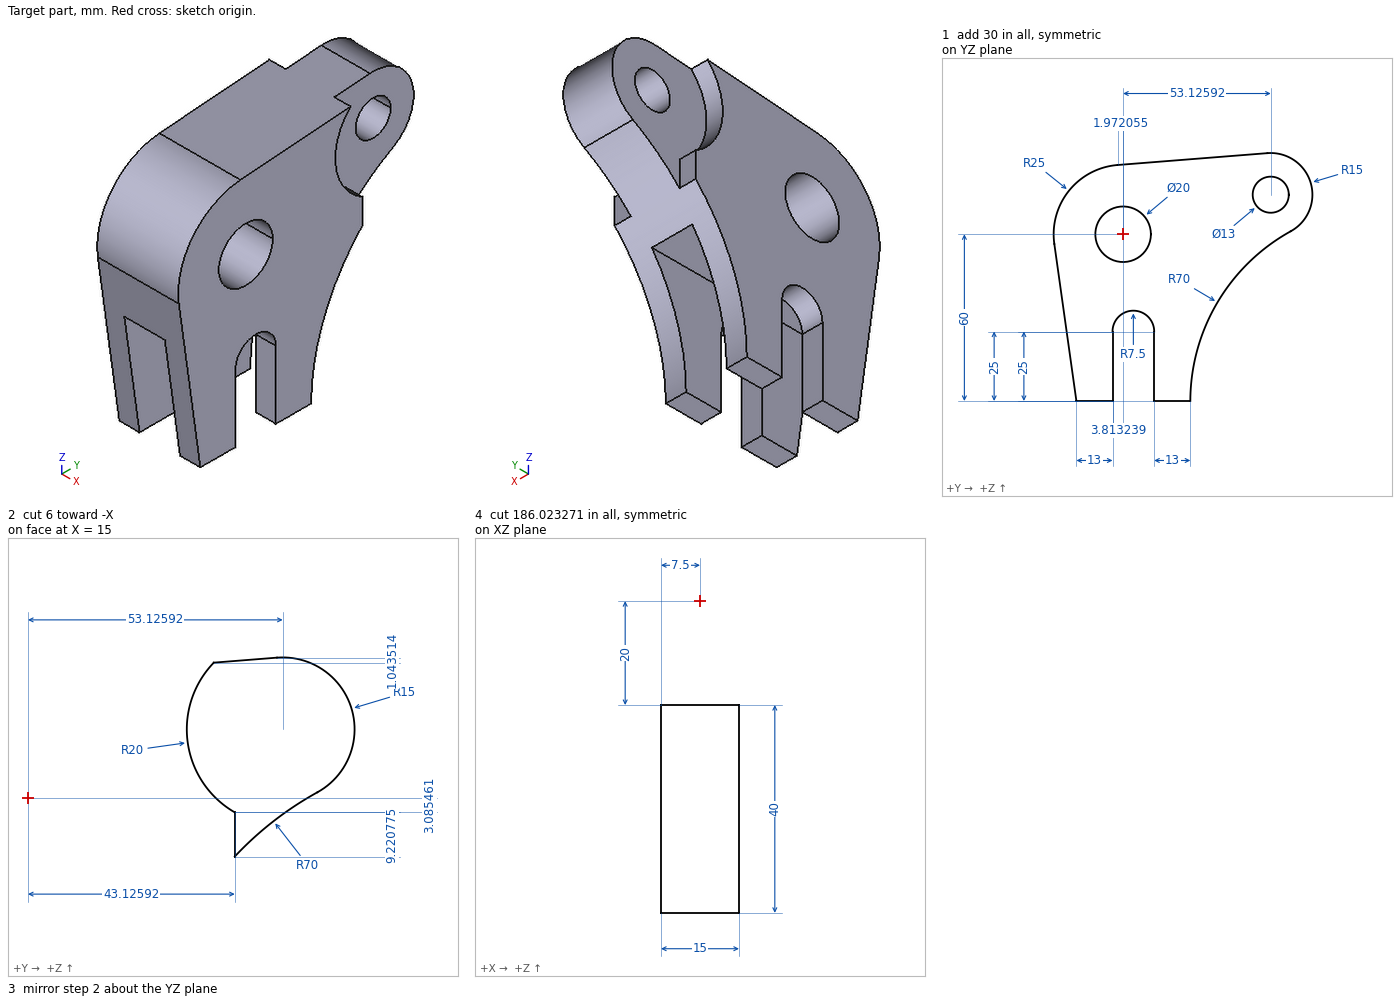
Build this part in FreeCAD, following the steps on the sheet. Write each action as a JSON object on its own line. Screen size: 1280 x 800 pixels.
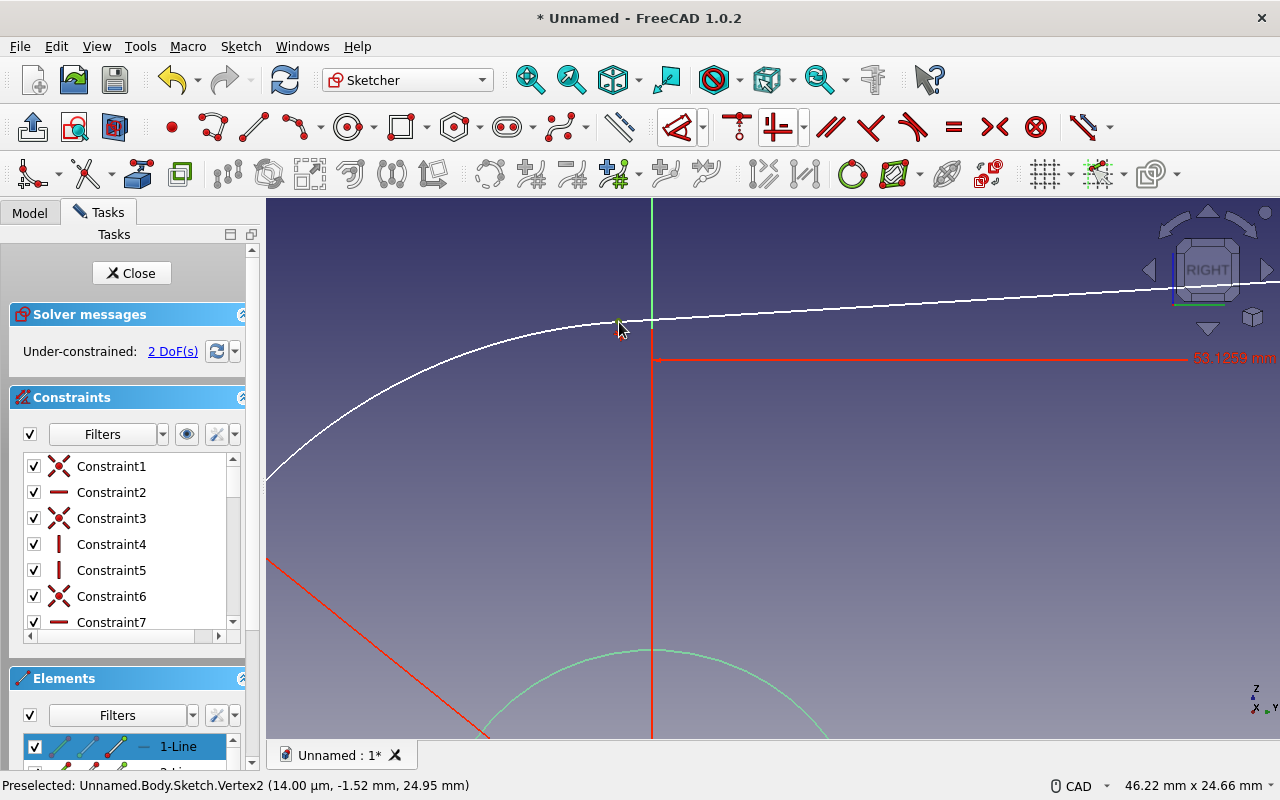
{"action": "left_click", "coordinate": [702, 128]}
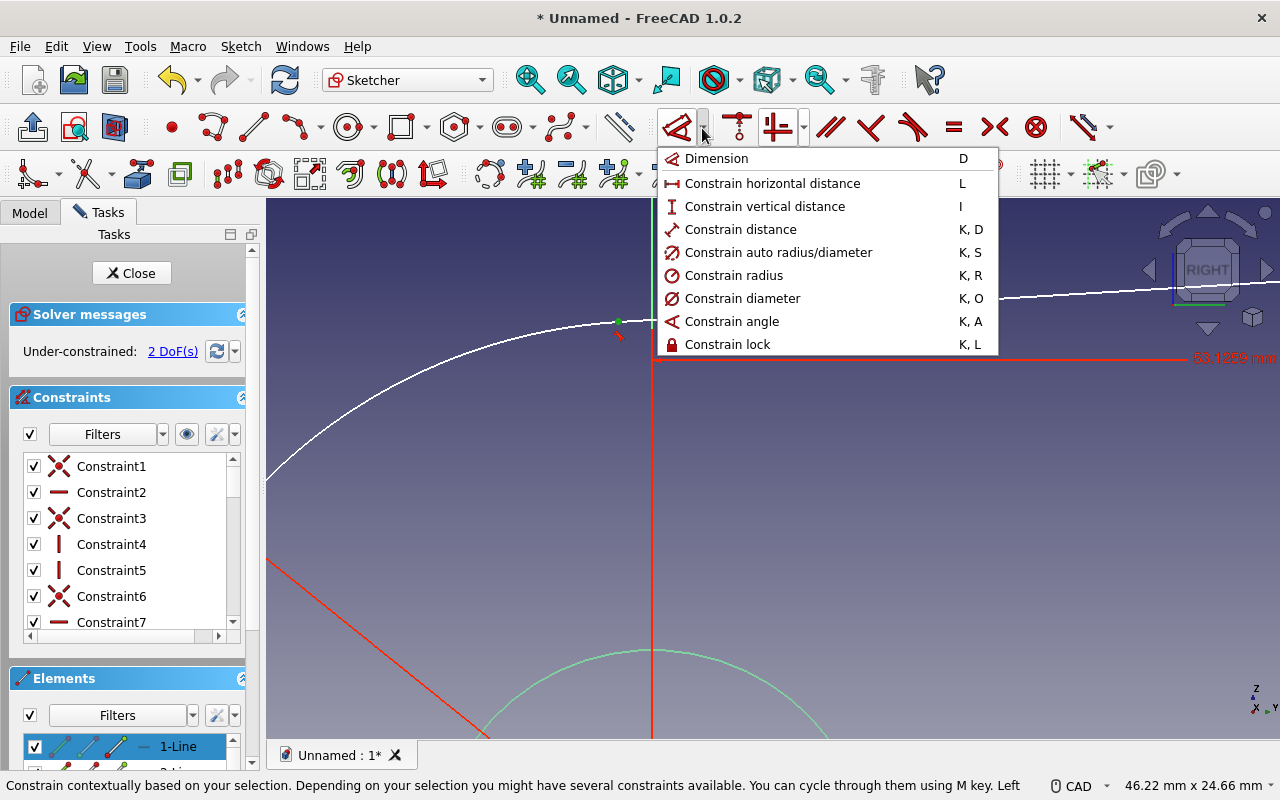
{"action": "left_click", "coordinate": [828, 184]}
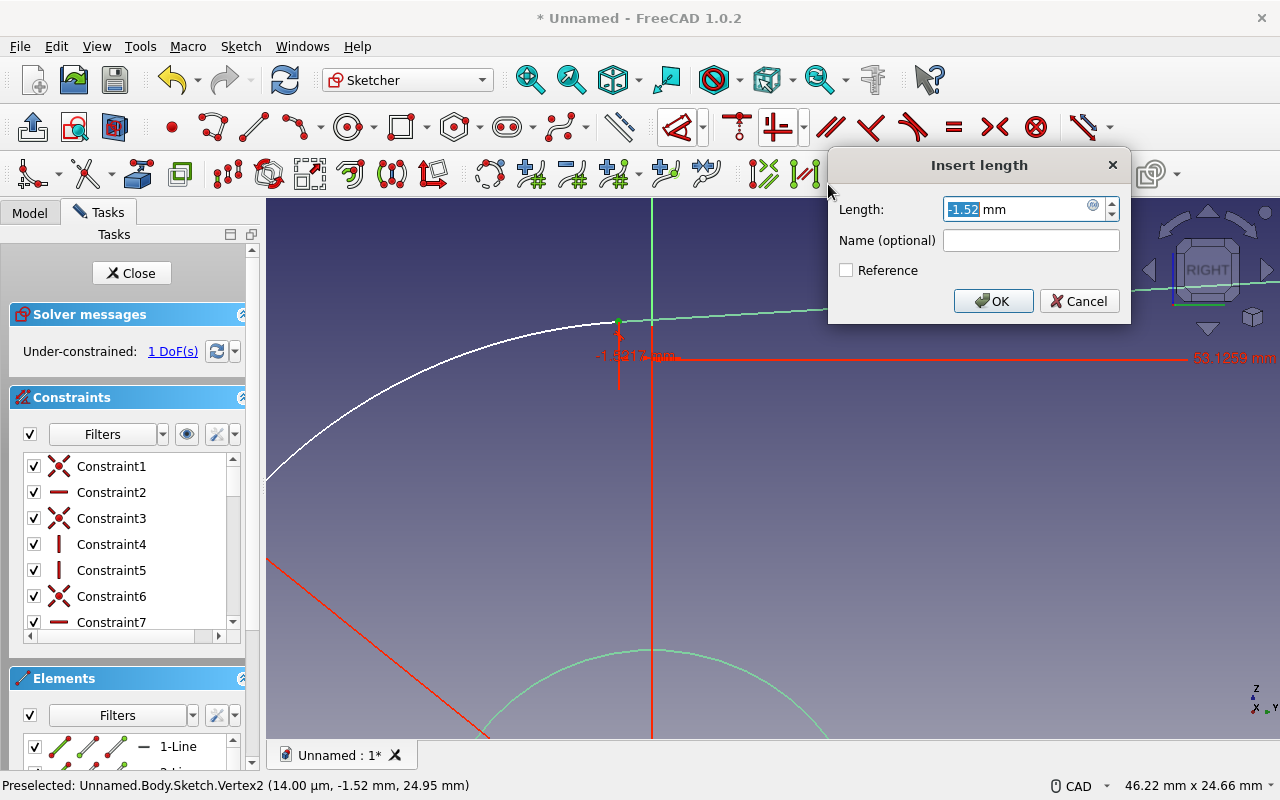
{"action": "type", "text": "-1.972055"}
{"action": "key", "text": "Return"}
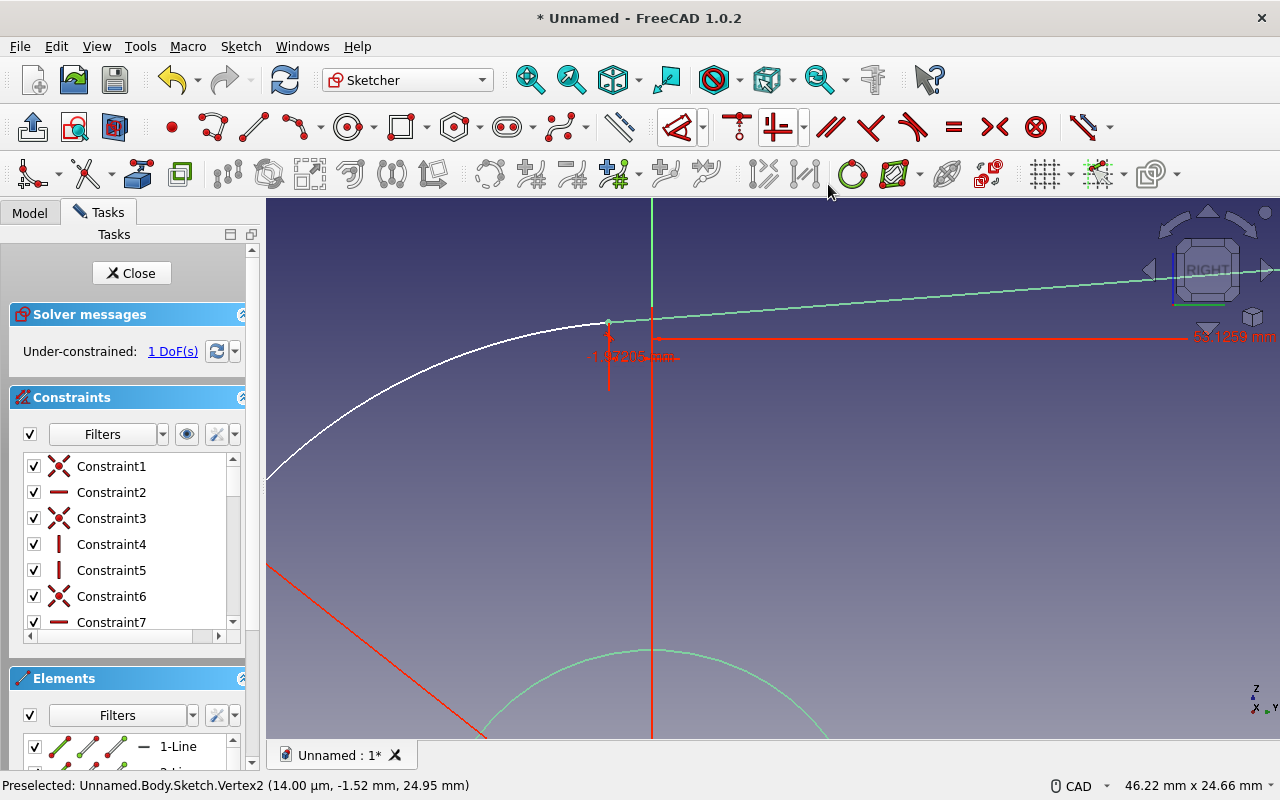
{"action": "scroll", "coordinate": [622, 322], "scroll_direction": "down", "scroll_amount": 9}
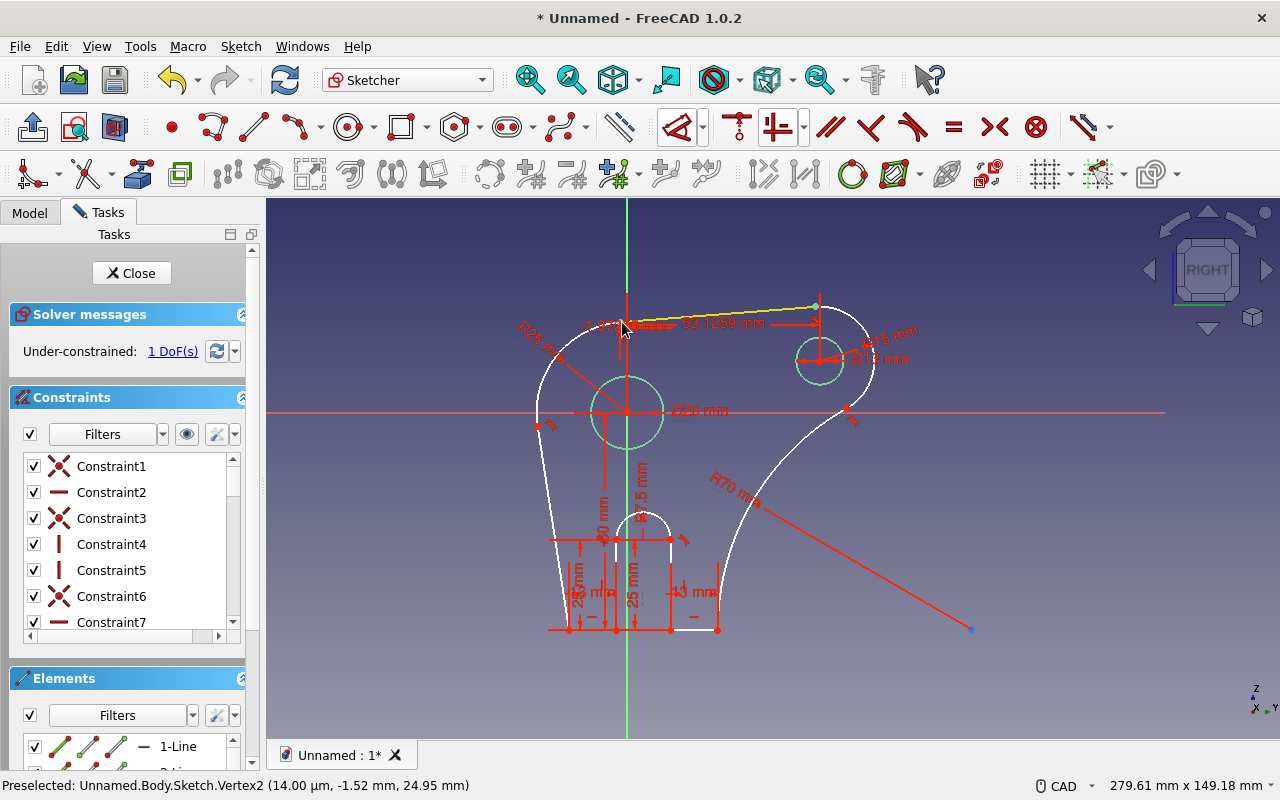
{"action": "scroll", "coordinate": [616, 630], "scroll_direction": "up", "scroll_amount": 6}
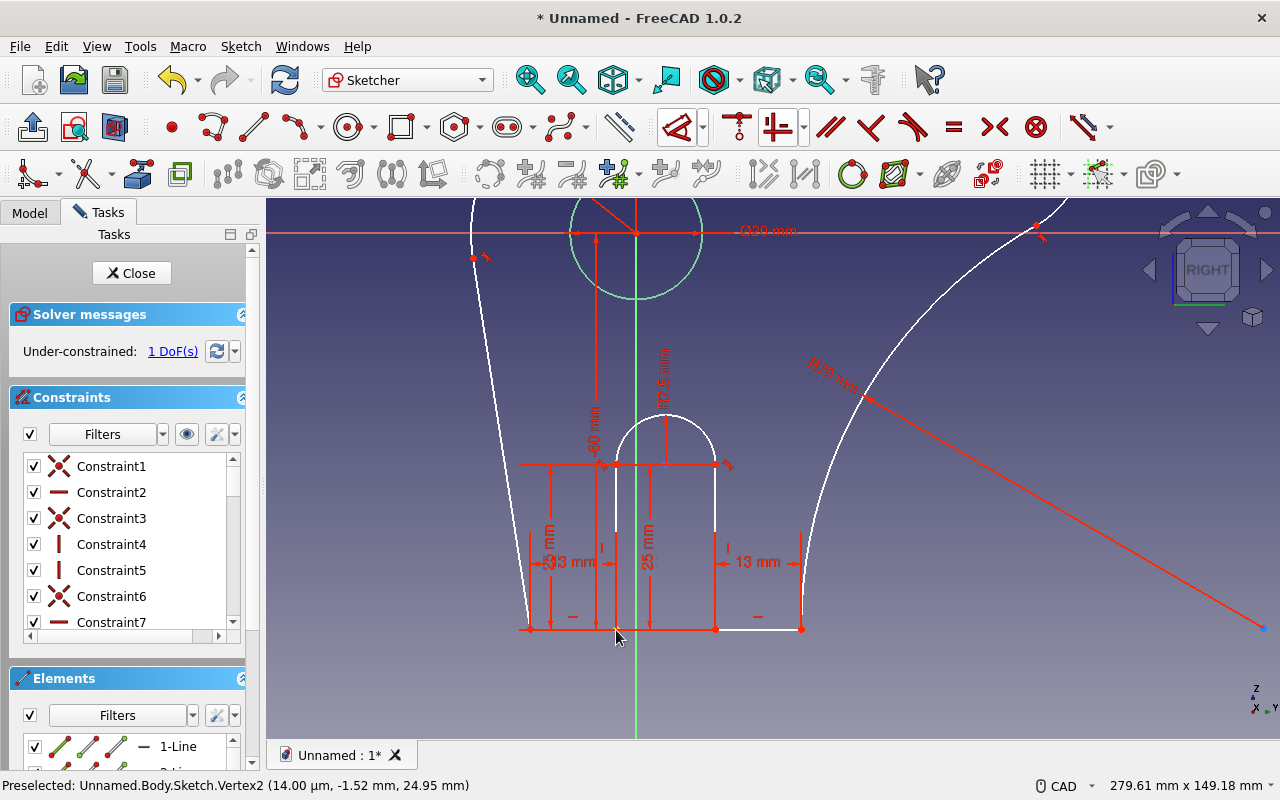
{"action": "left_click", "coordinate": [616, 629]}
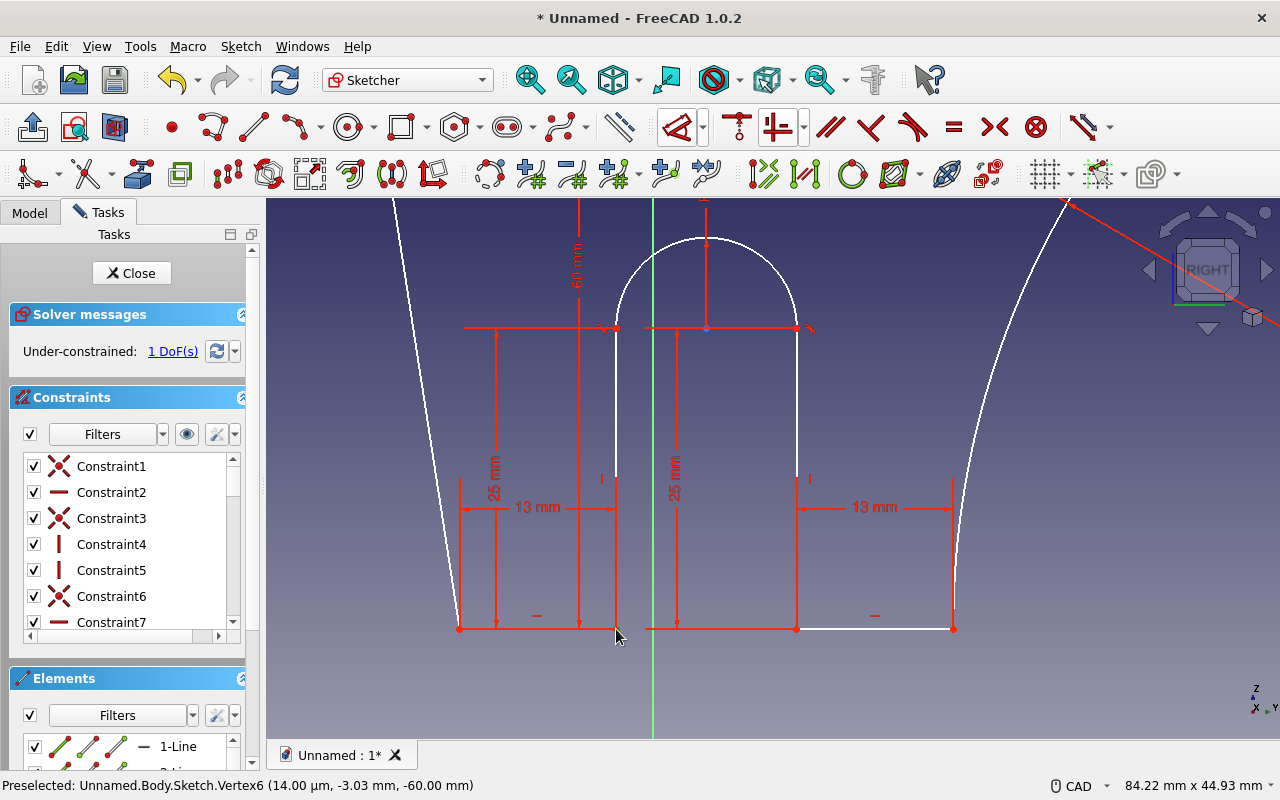
{"action": "left_click", "coordinate": [702, 128]}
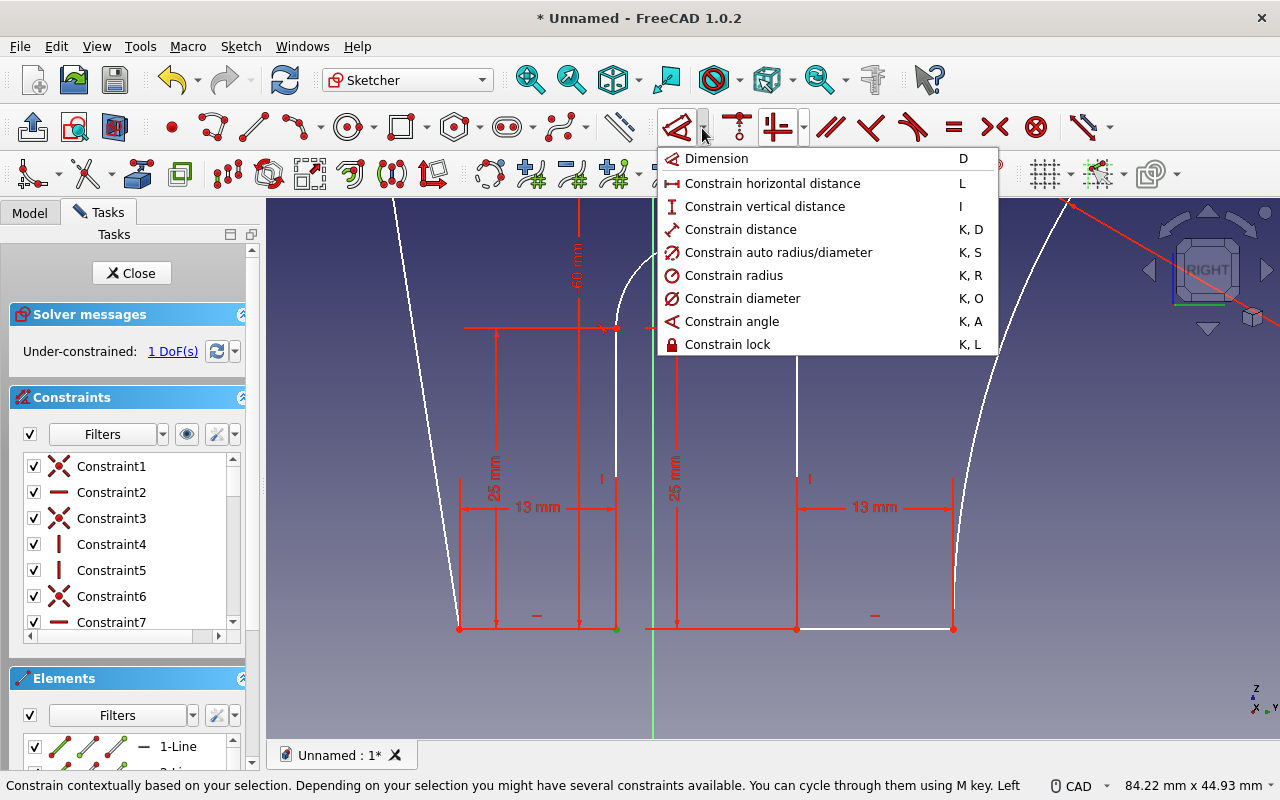
{"action": "left_click", "coordinate": [828, 184]}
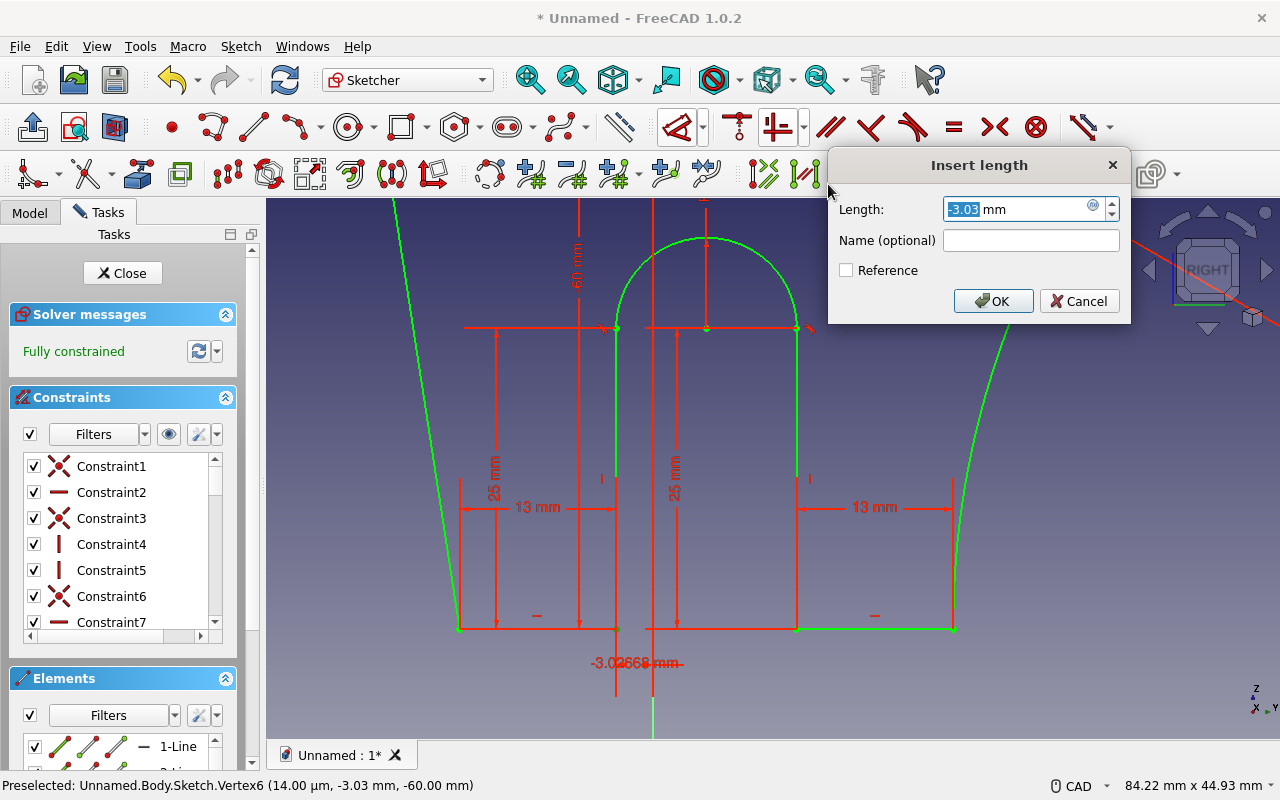
{"action": "type", "text": "-3.813239"}
{"action": "key", "text": "Return"}